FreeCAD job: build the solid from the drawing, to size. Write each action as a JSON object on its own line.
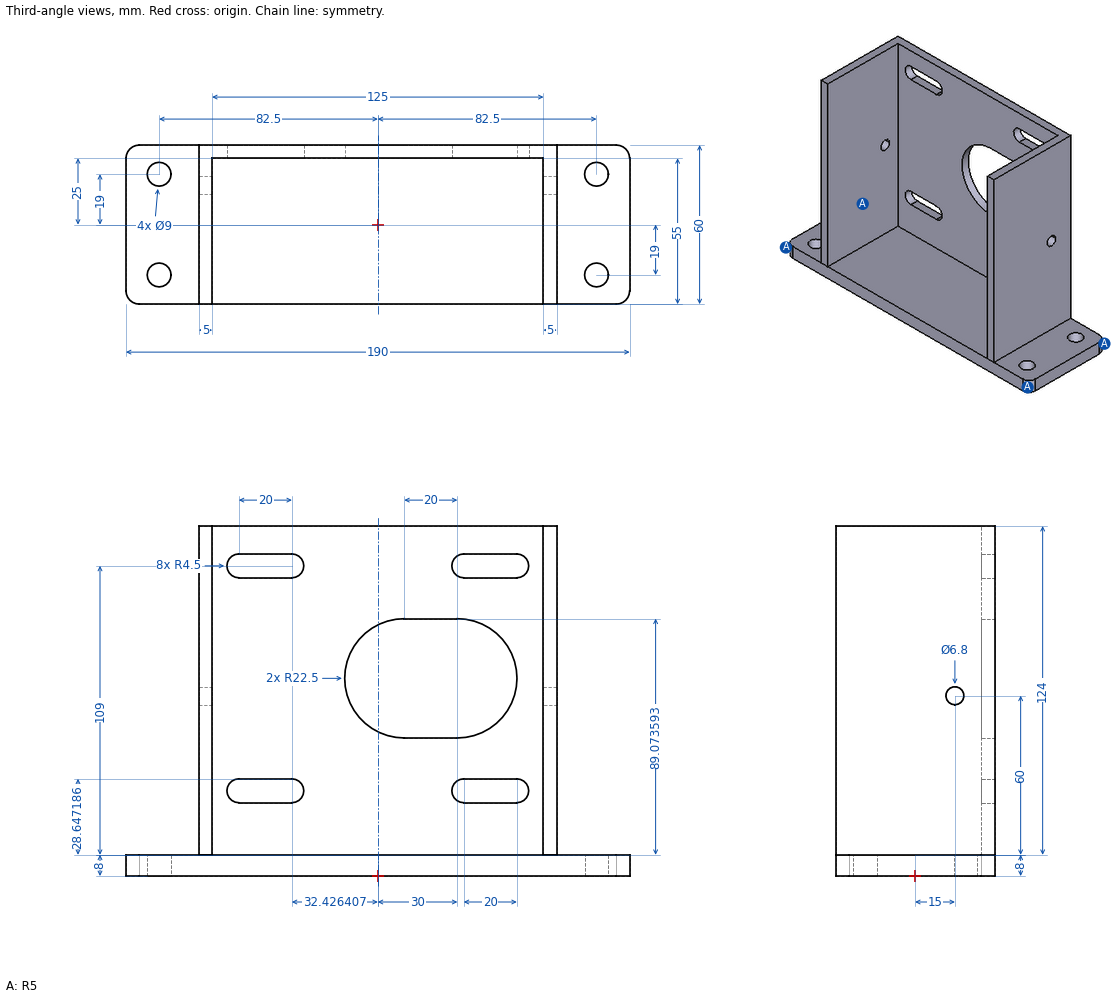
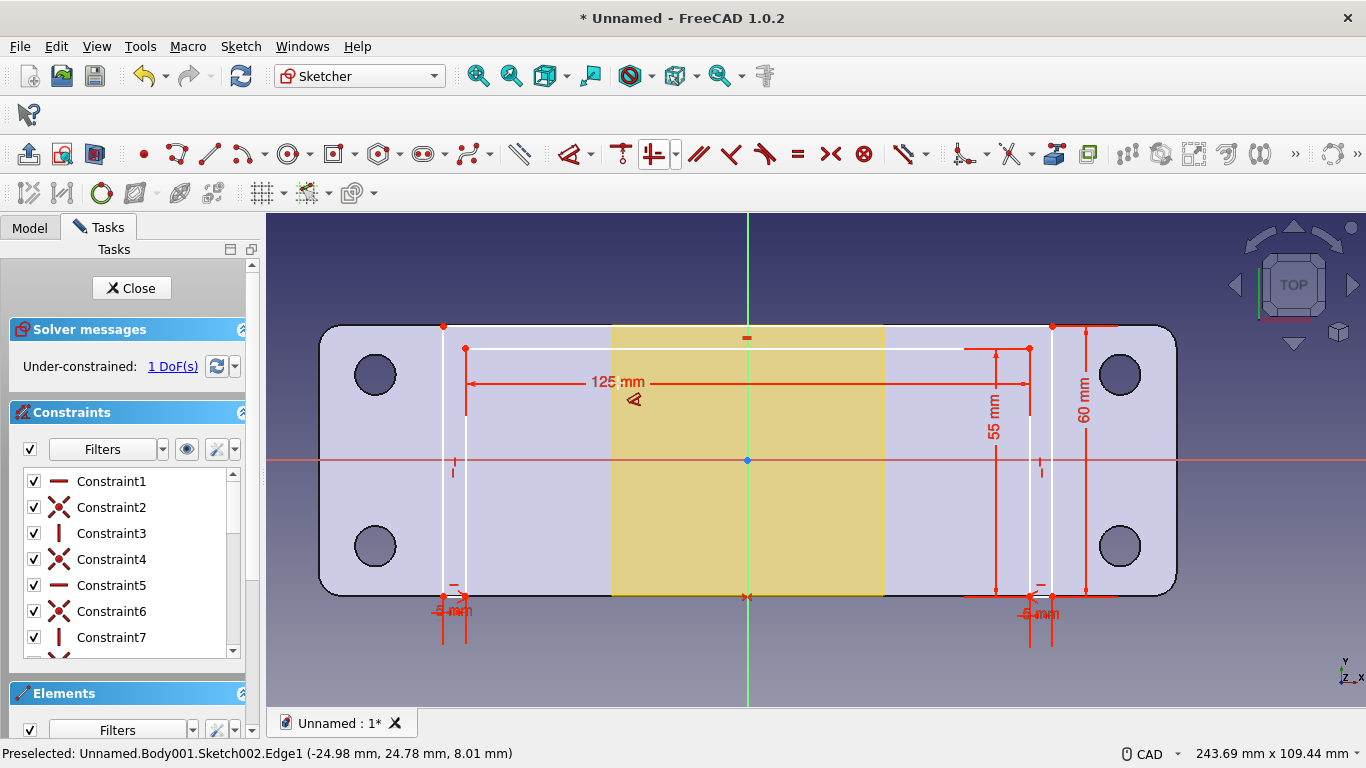
{"action": "left_click", "coordinate": [466, 349]}
{"action": "left_click", "coordinate": [782, 405]}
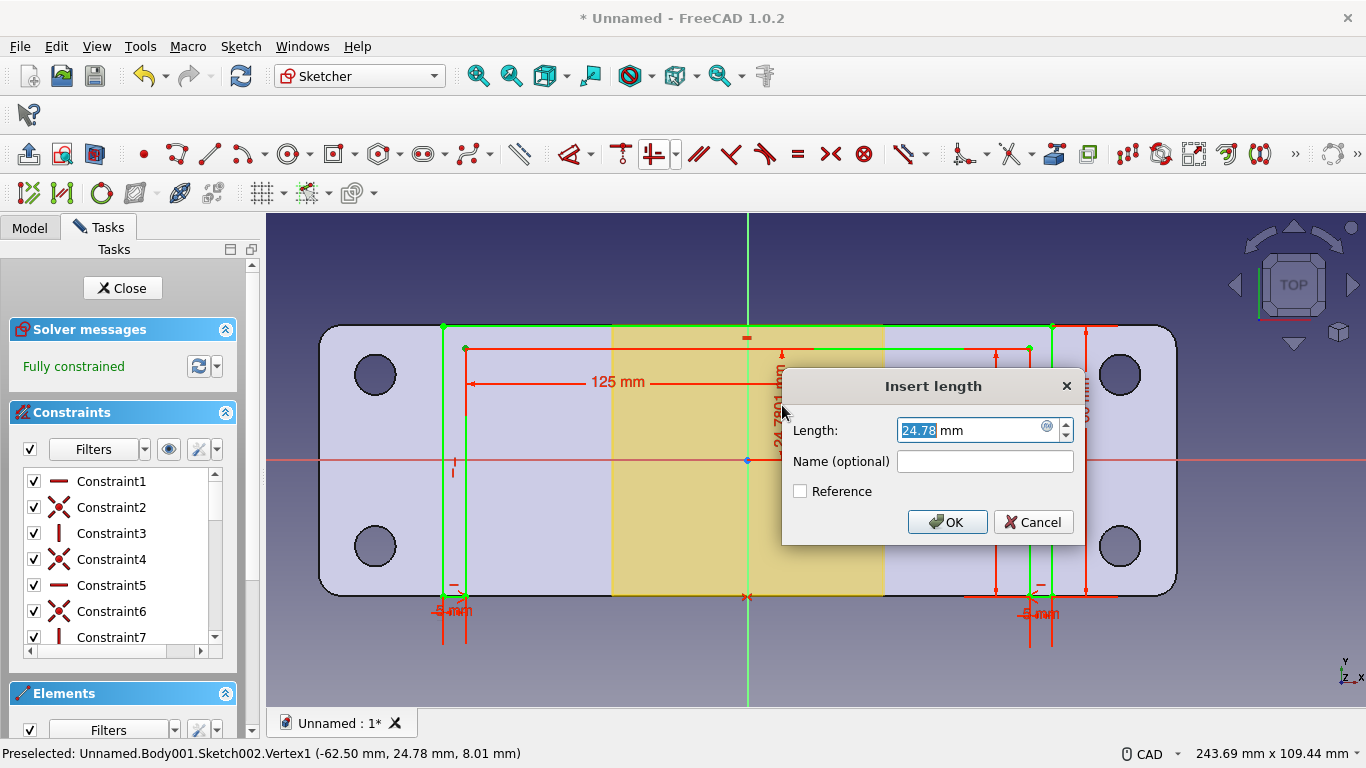
{"action": "type", "text": "25"}
{"action": "key", "text": "Return"}
{"action": "key", "text": "Escape"}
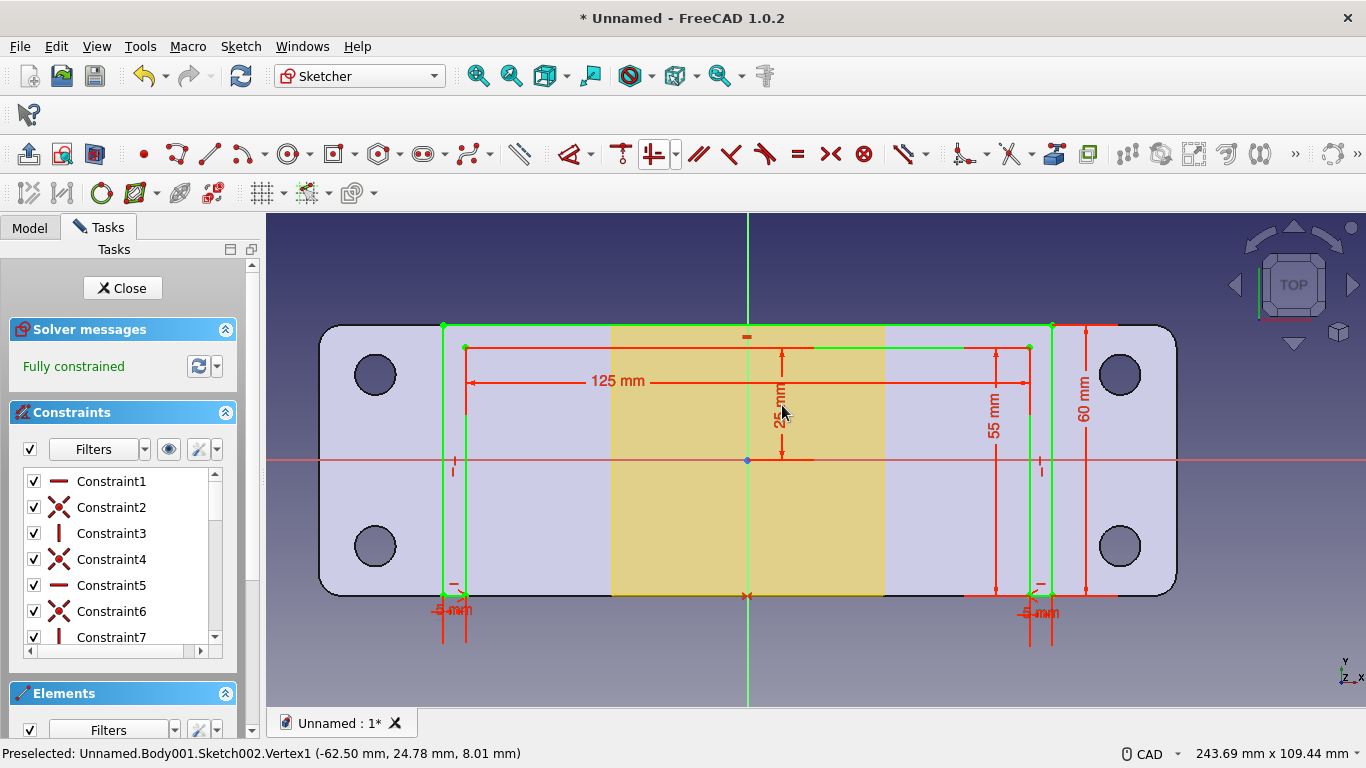
{"action": "left_click", "coordinate": [123, 288]}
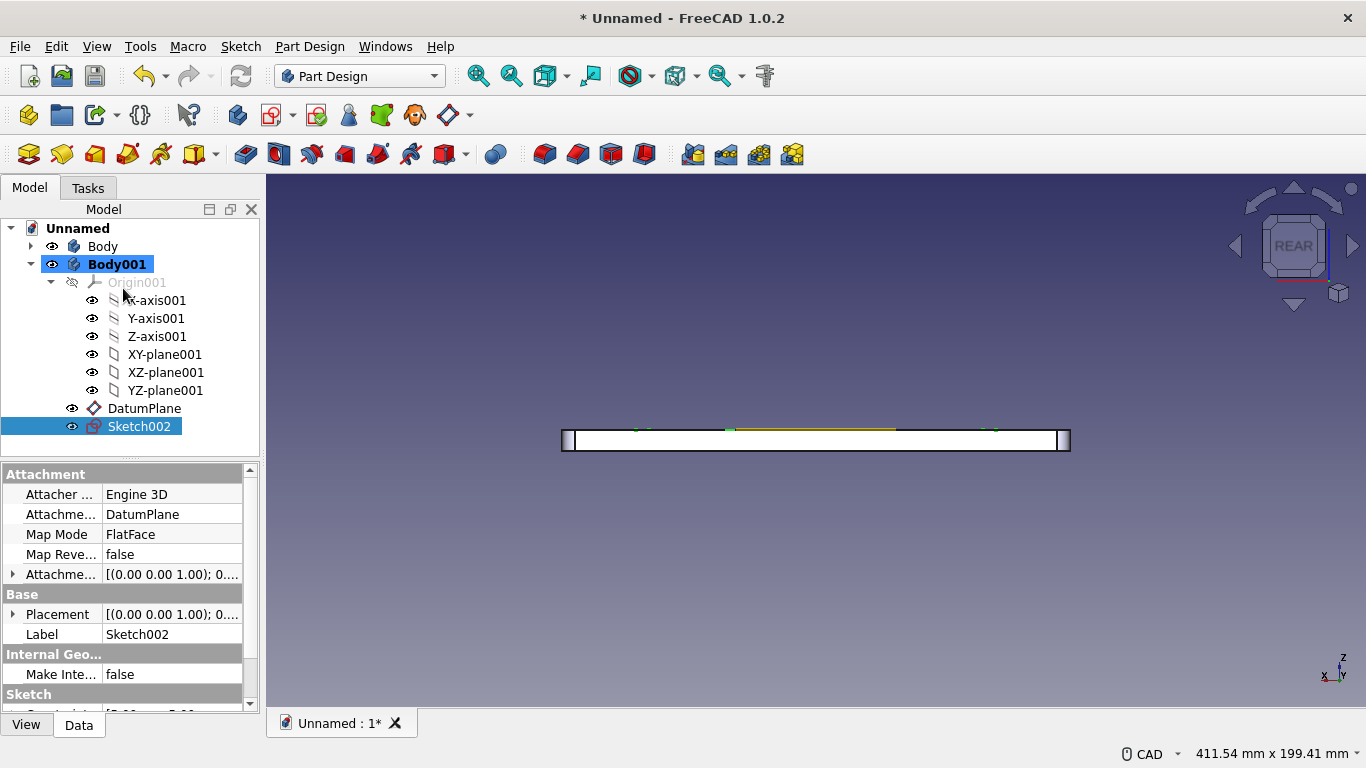
{"action": "left_click", "coordinate": [29, 154]}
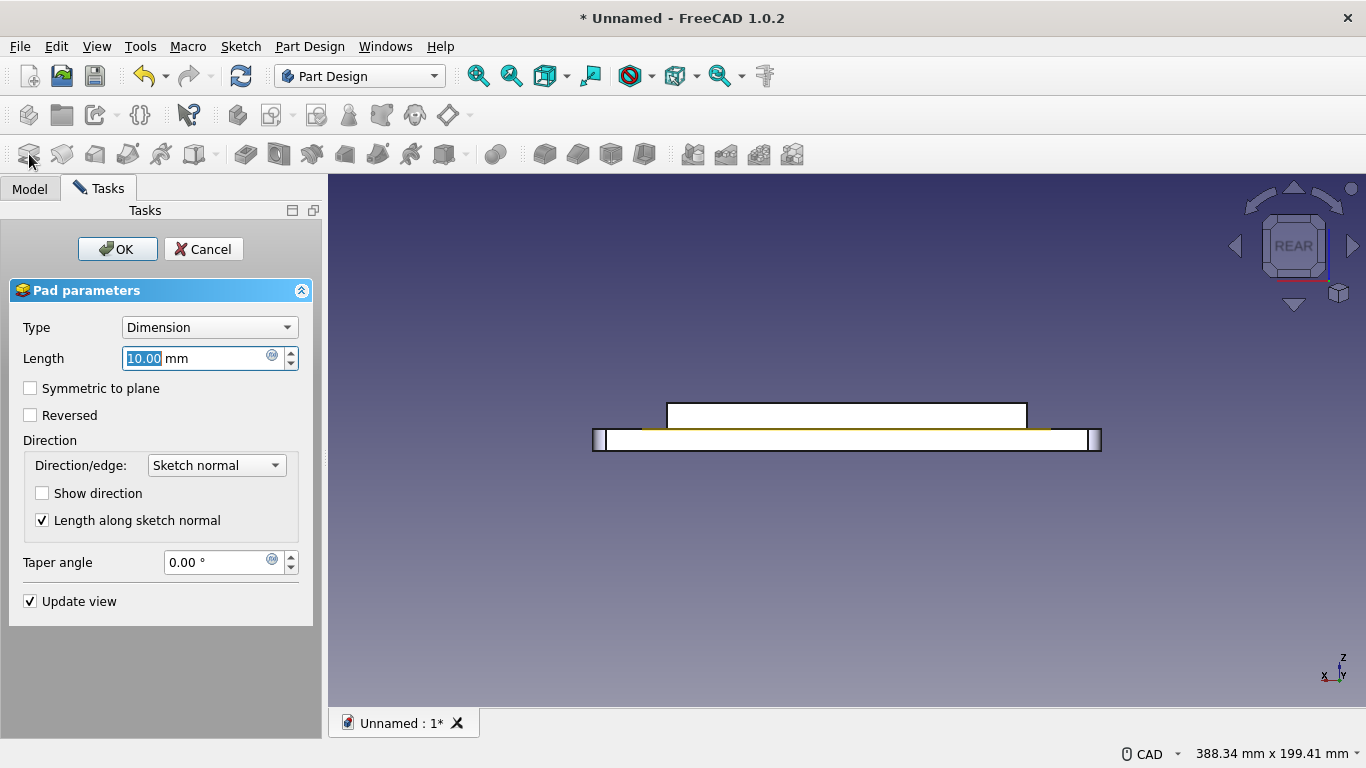
{"action": "type", "text": "124"}
{"action": "key", "text": "Tab"}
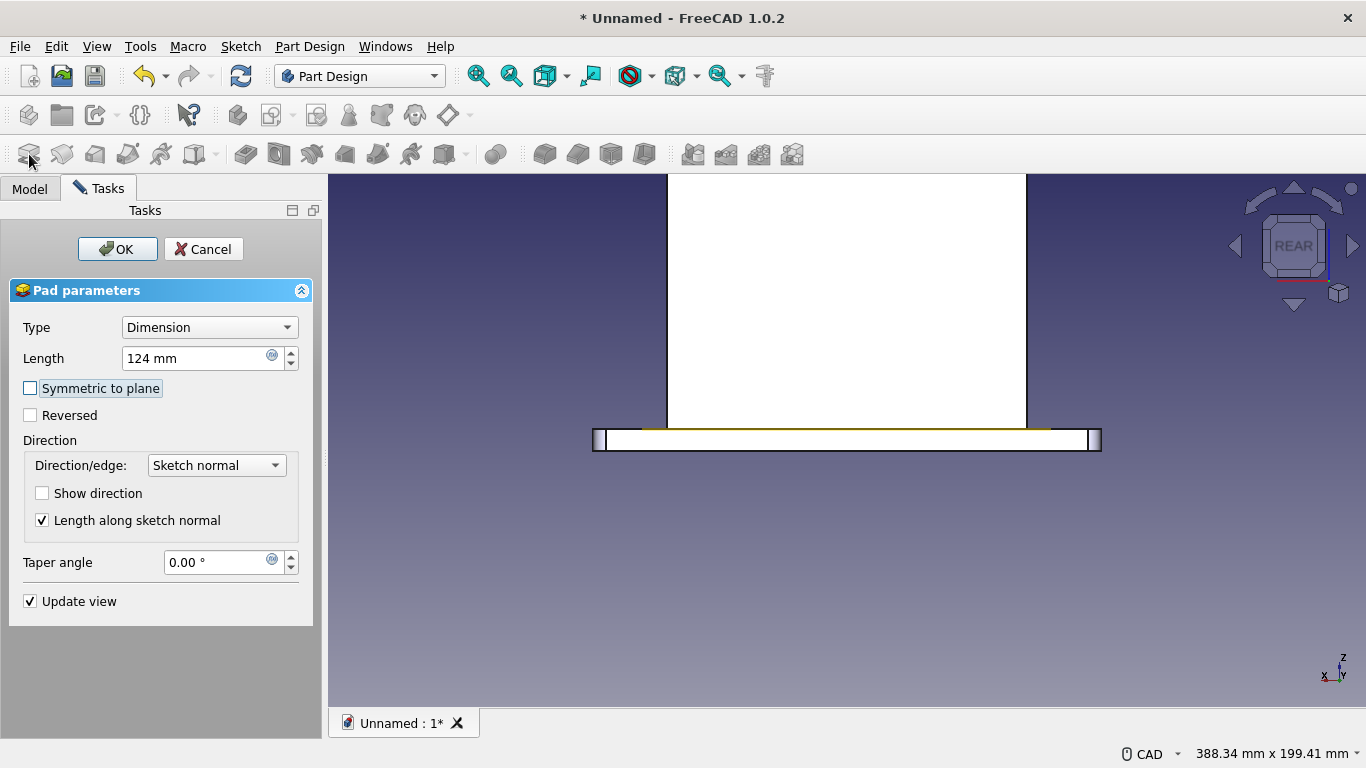
{"action": "left_click", "coordinate": [118, 249]}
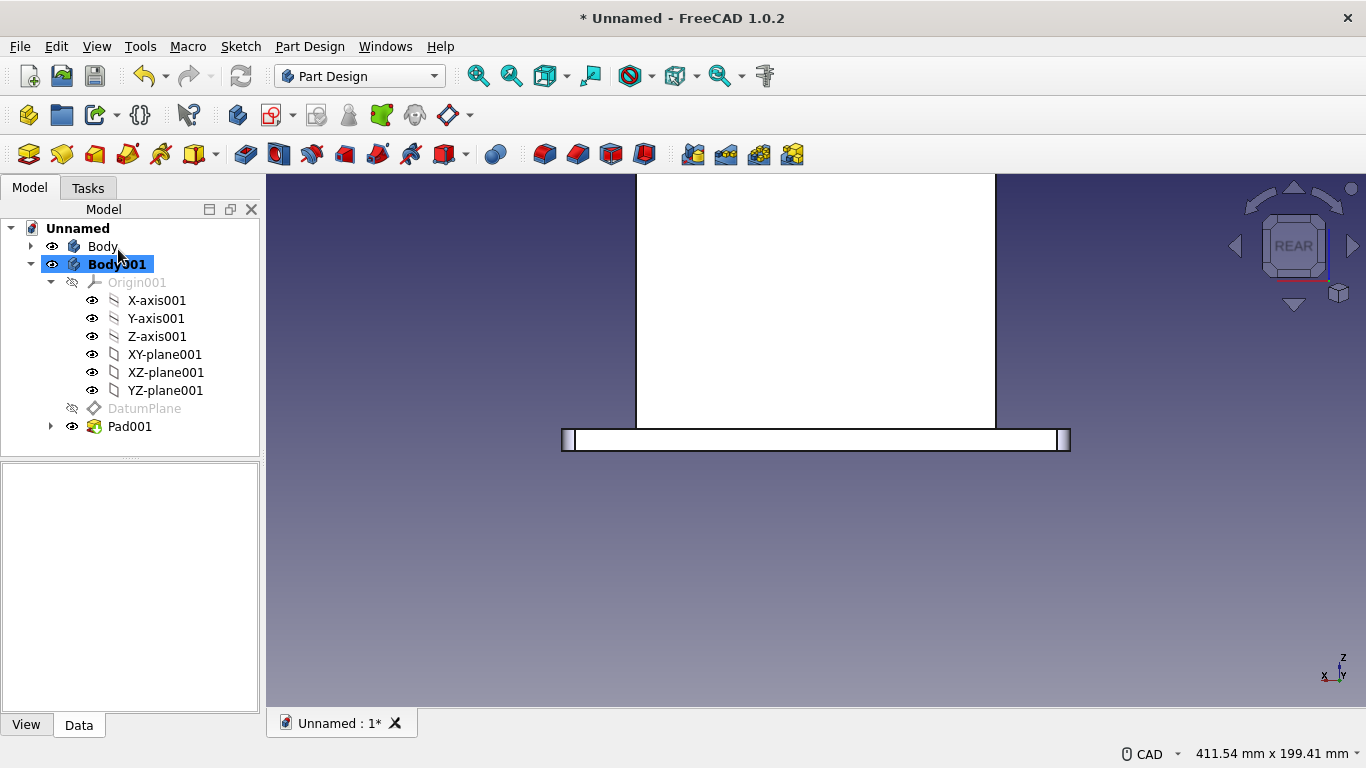
{"action": "left_click", "coordinate": [479, 76]}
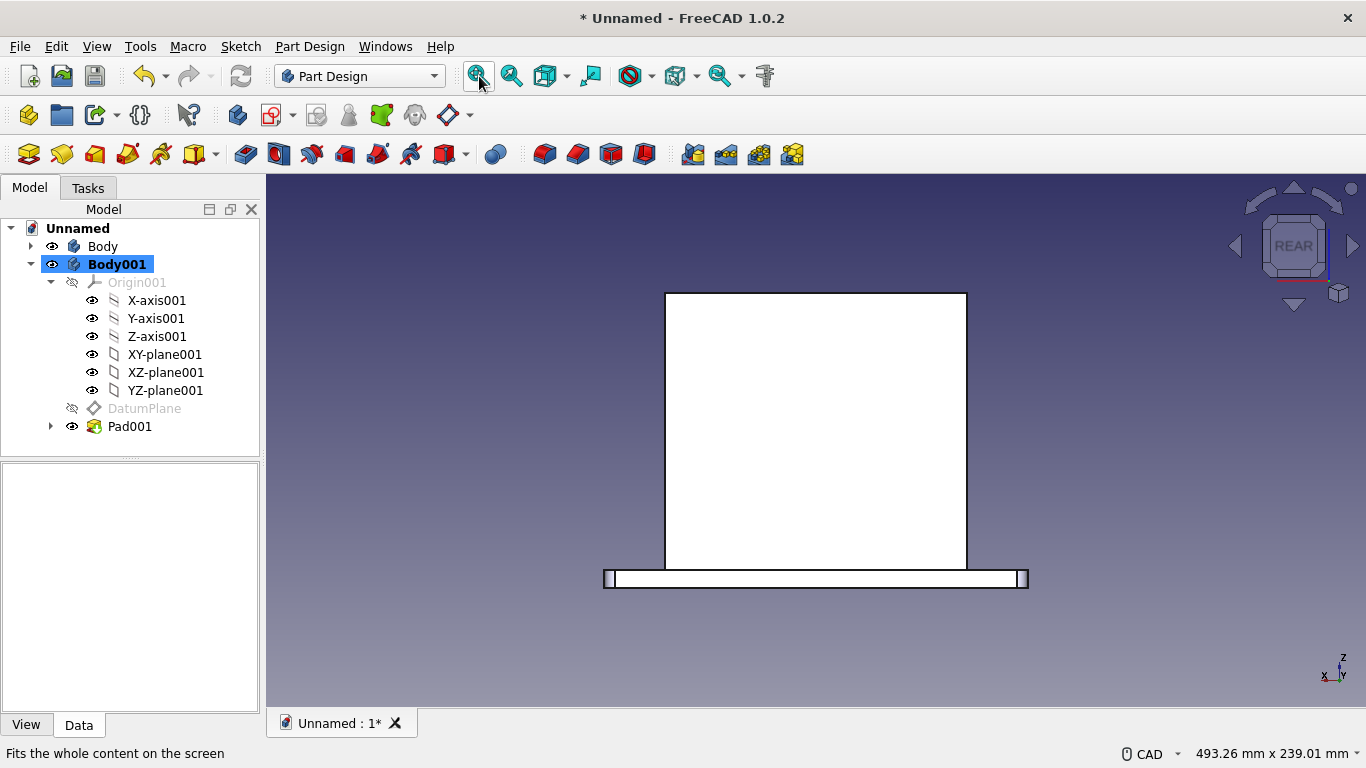
{"action": "left_click", "coordinate": [816, 431]}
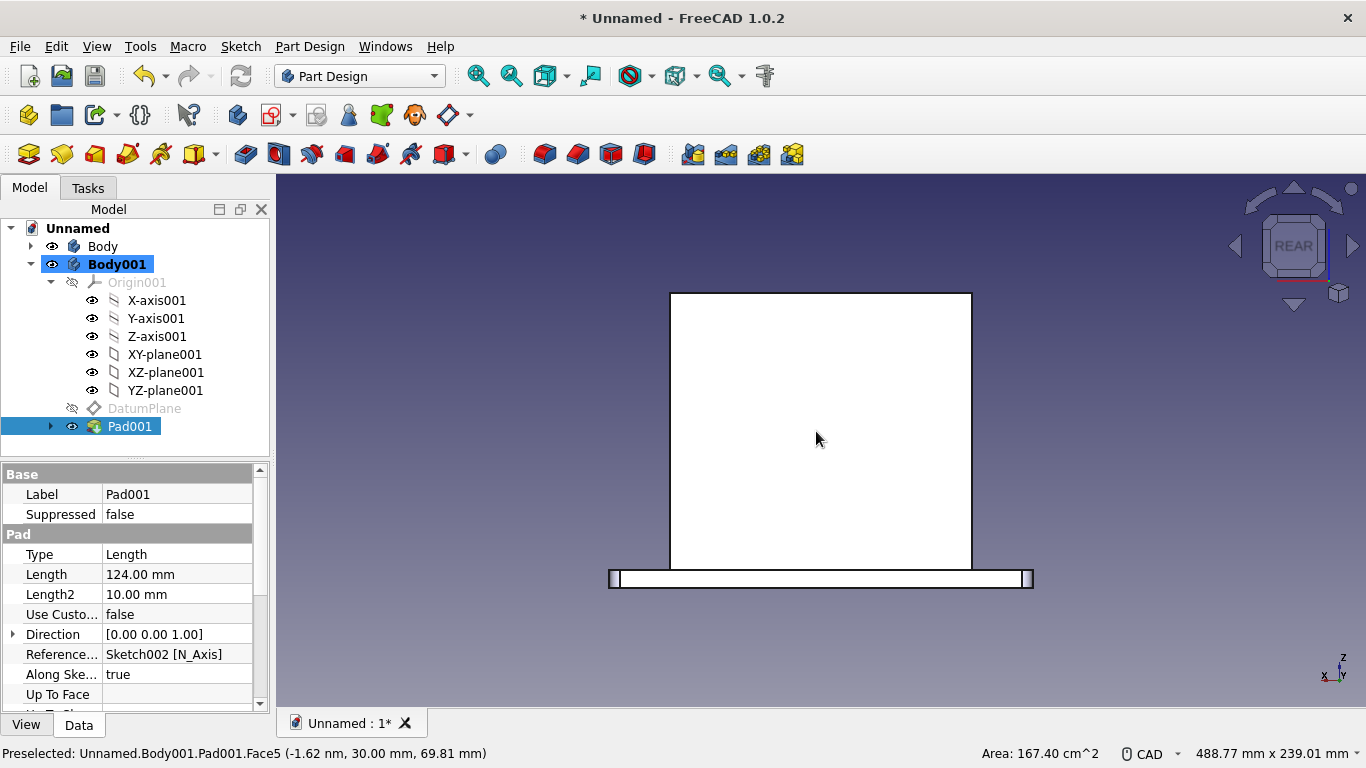
{"action": "left_click", "coordinate": [270, 116]}